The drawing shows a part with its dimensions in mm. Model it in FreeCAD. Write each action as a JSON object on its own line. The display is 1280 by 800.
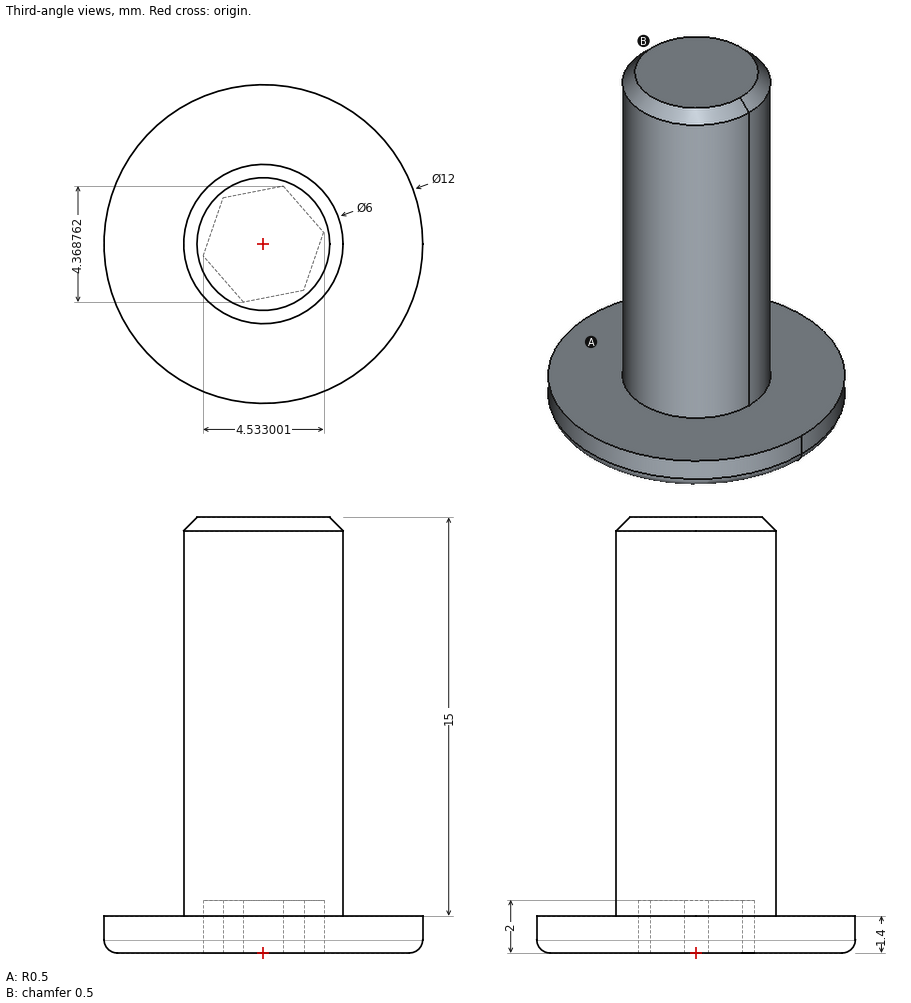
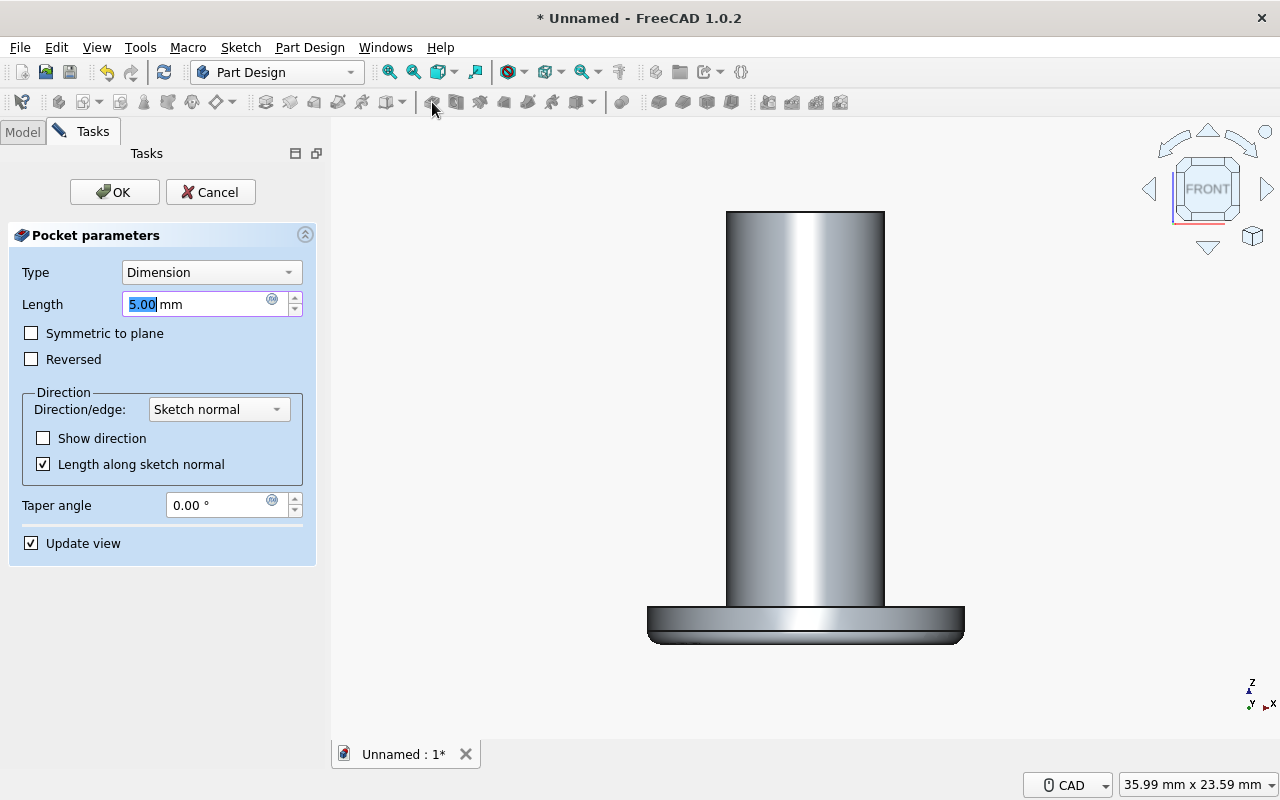
{"action": "type", "text": "2"}
{"action": "key", "text": "Tab"}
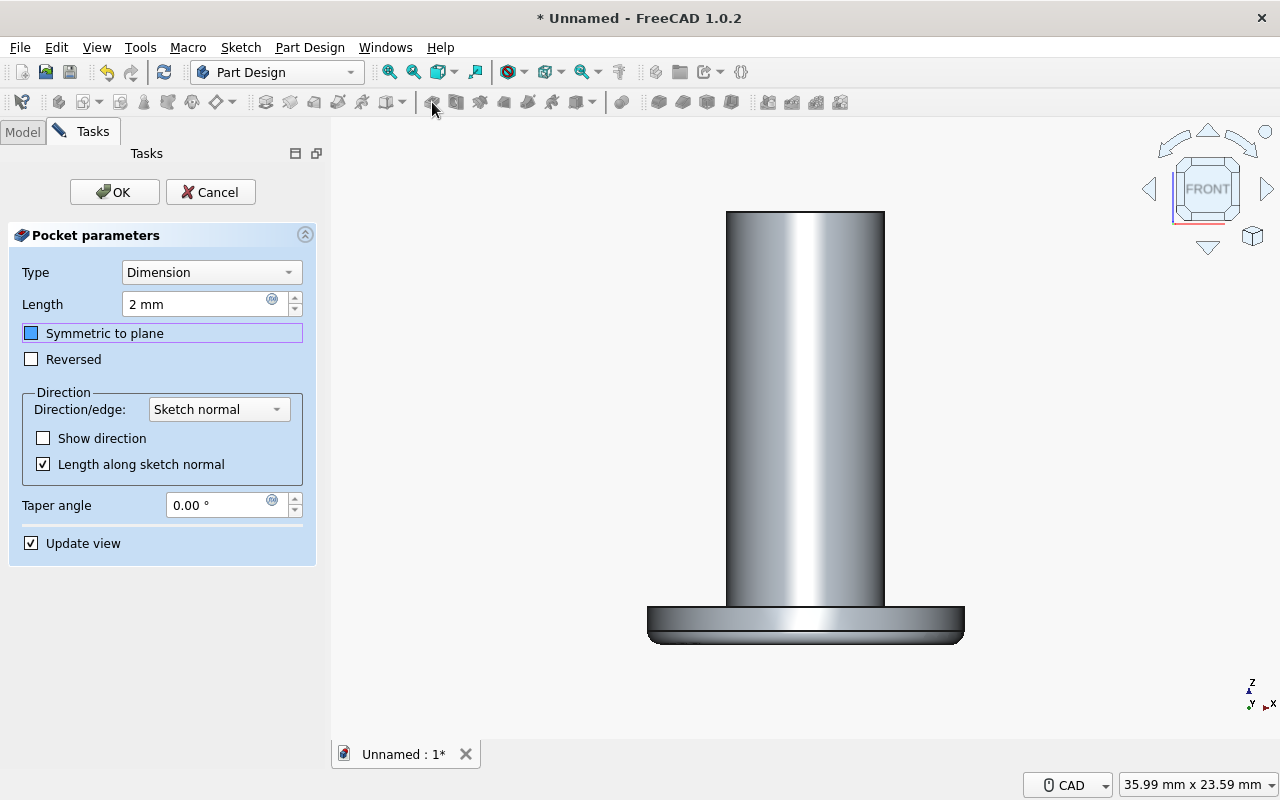
{"action": "left_click", "coordinate": [30, 359]}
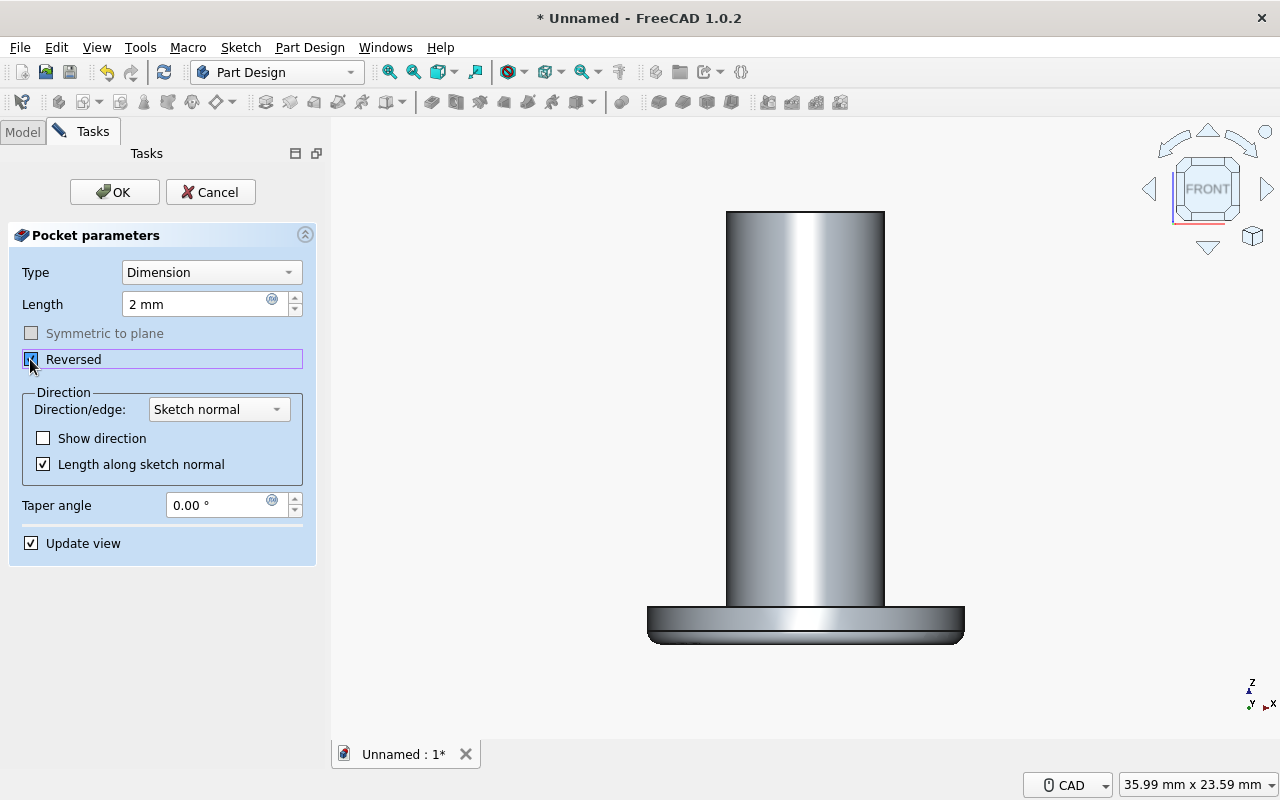
{"action": "left_click", "coordinate": [115, 192]}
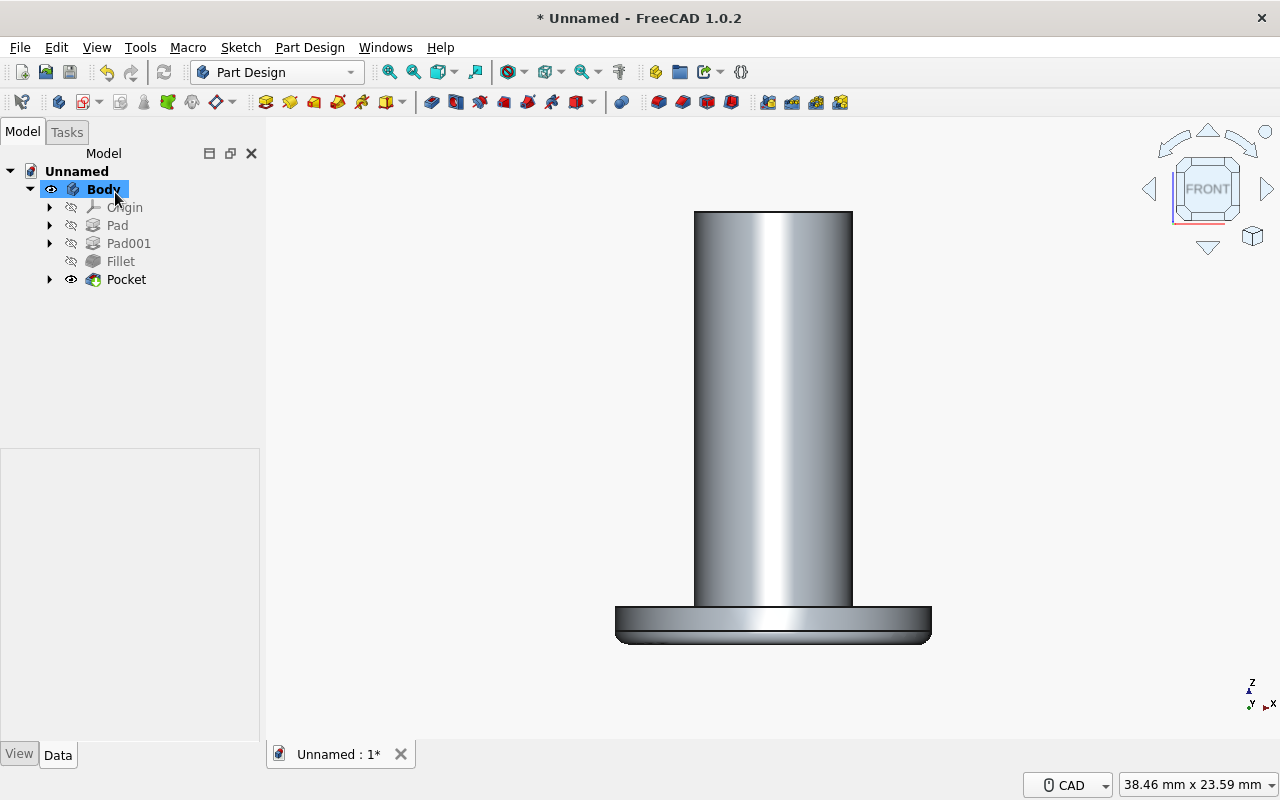
{"action": "left_click", "coordinate": [709, 211]}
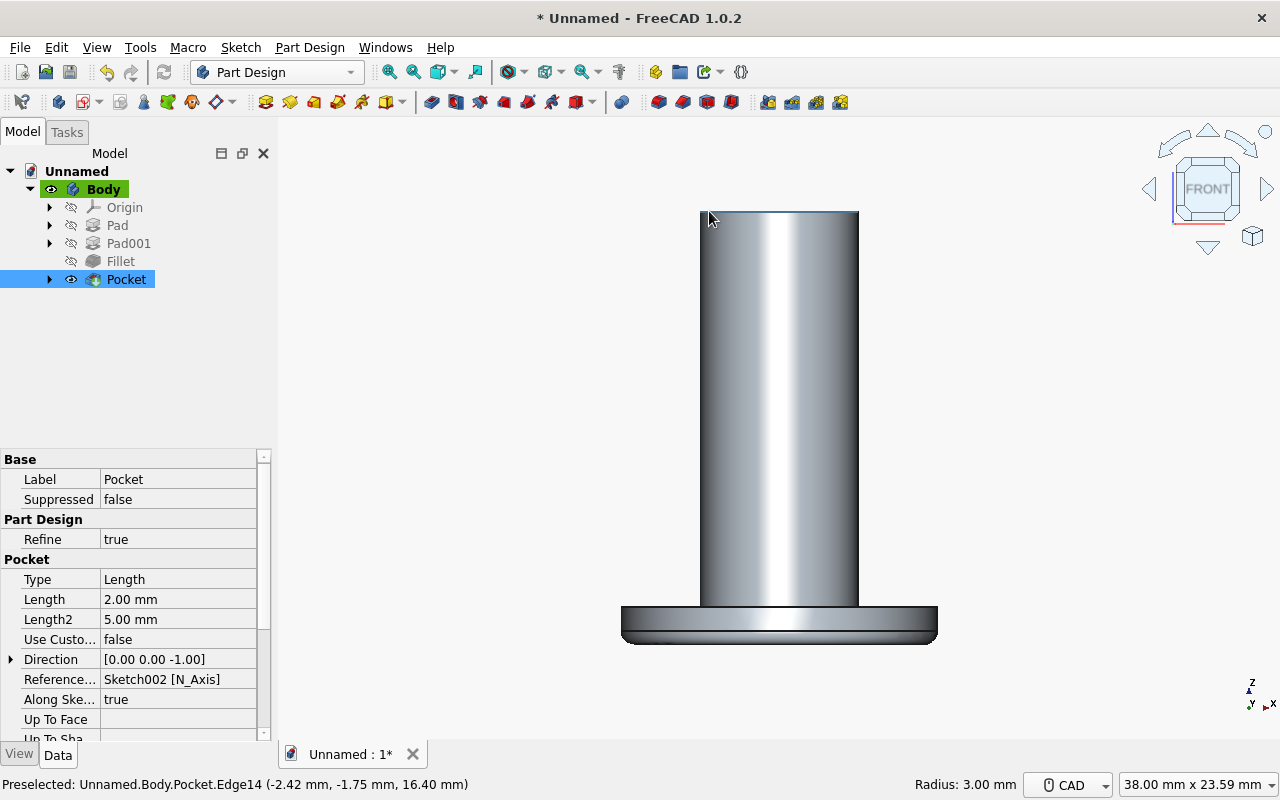
{"action": "left_click", "coordinate": [684, 102]}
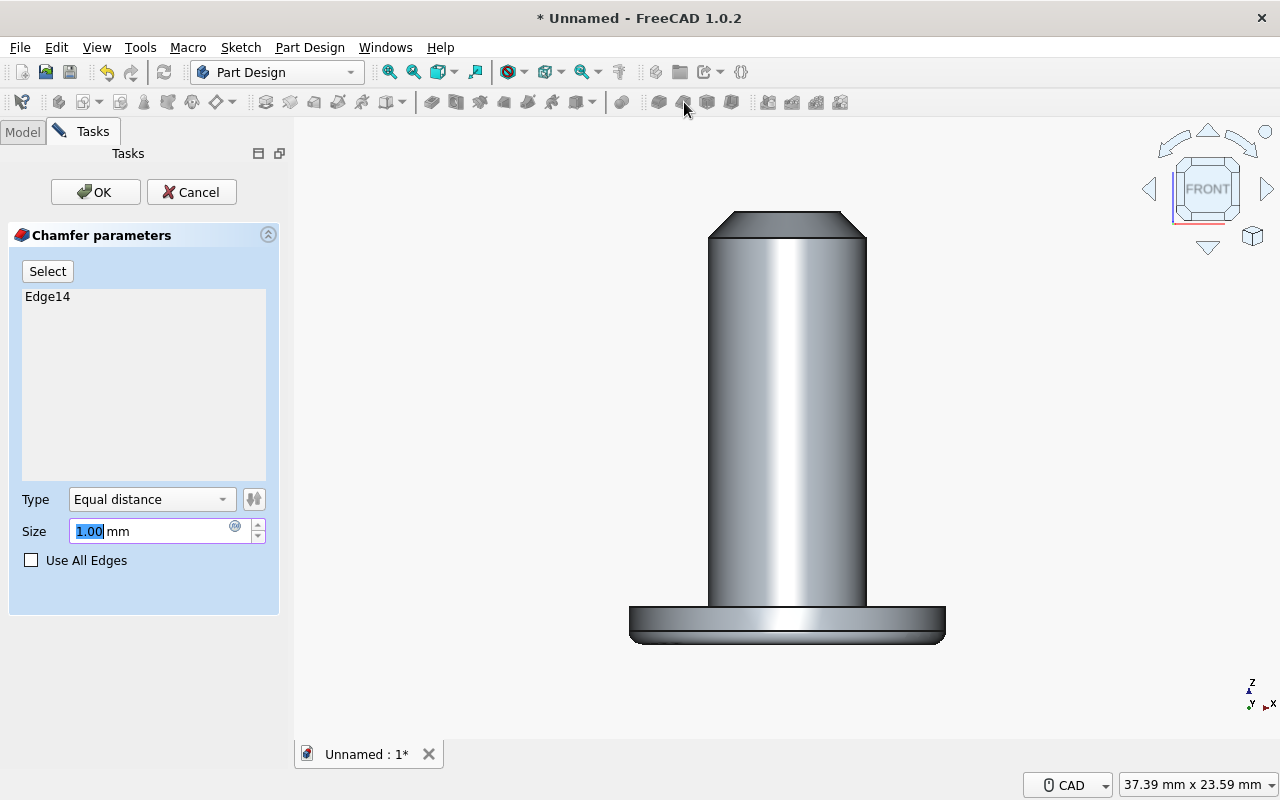
{"action": "type", "text": "0.5"}
{"action": "key", "text": "Tab"}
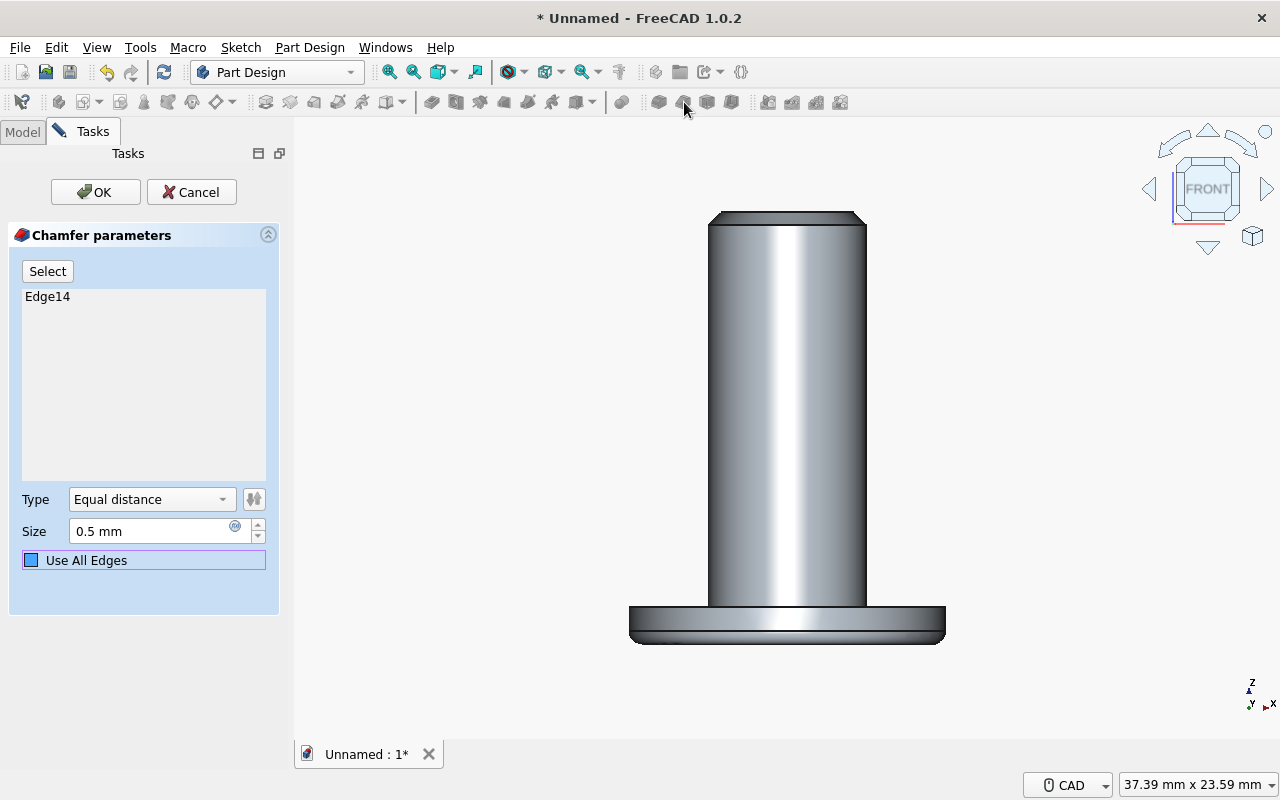
{"action": "left_click", "coordinate": [96, 192]}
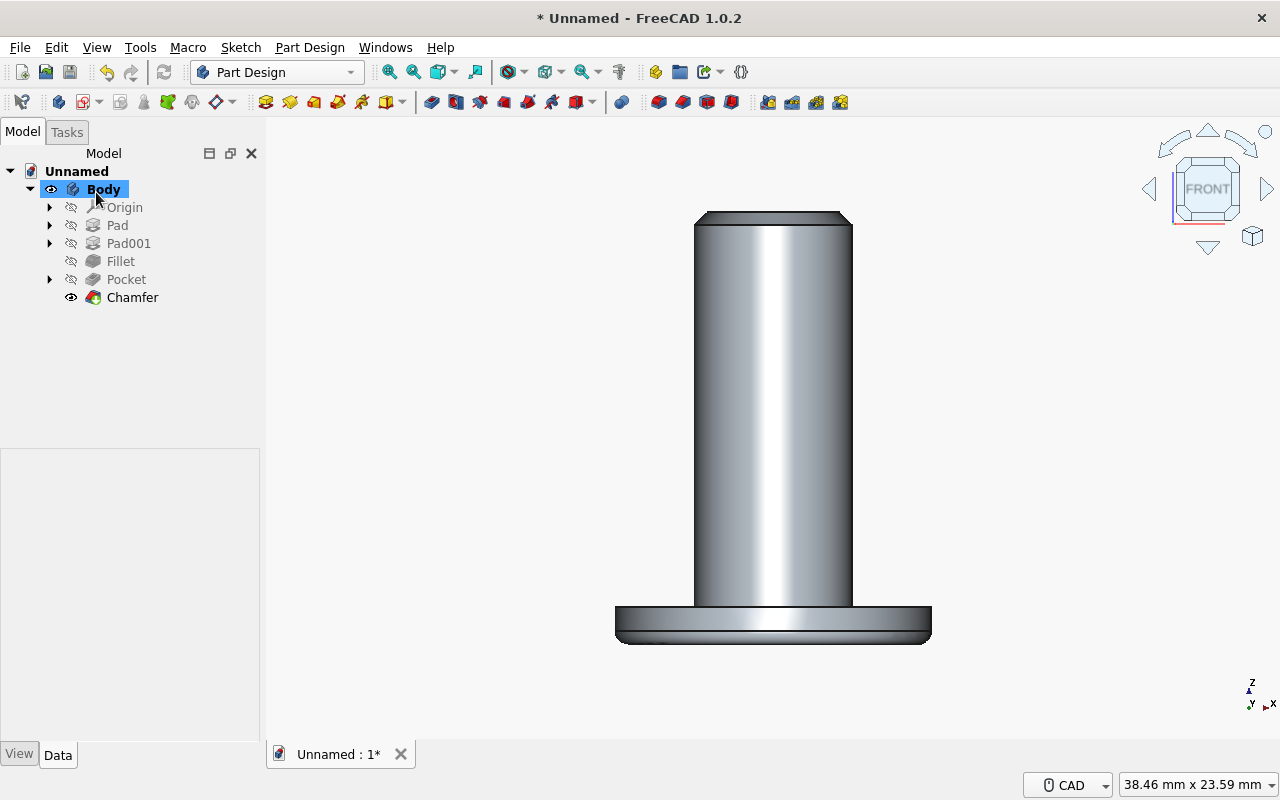
{"action": "key", "text": "0"}